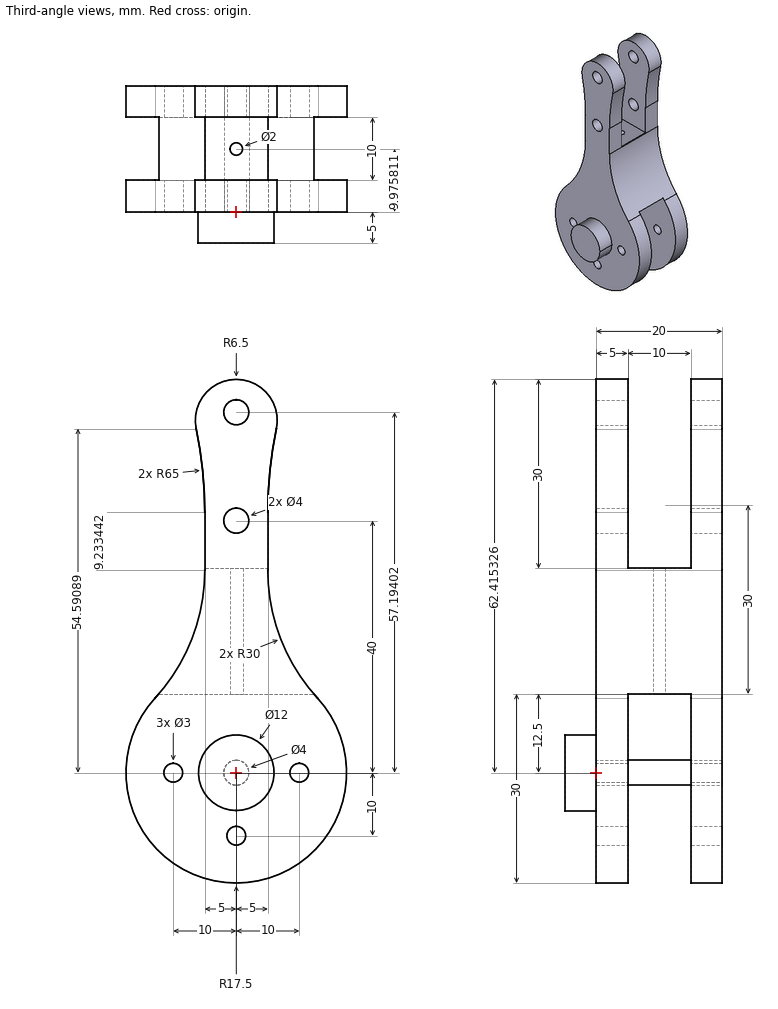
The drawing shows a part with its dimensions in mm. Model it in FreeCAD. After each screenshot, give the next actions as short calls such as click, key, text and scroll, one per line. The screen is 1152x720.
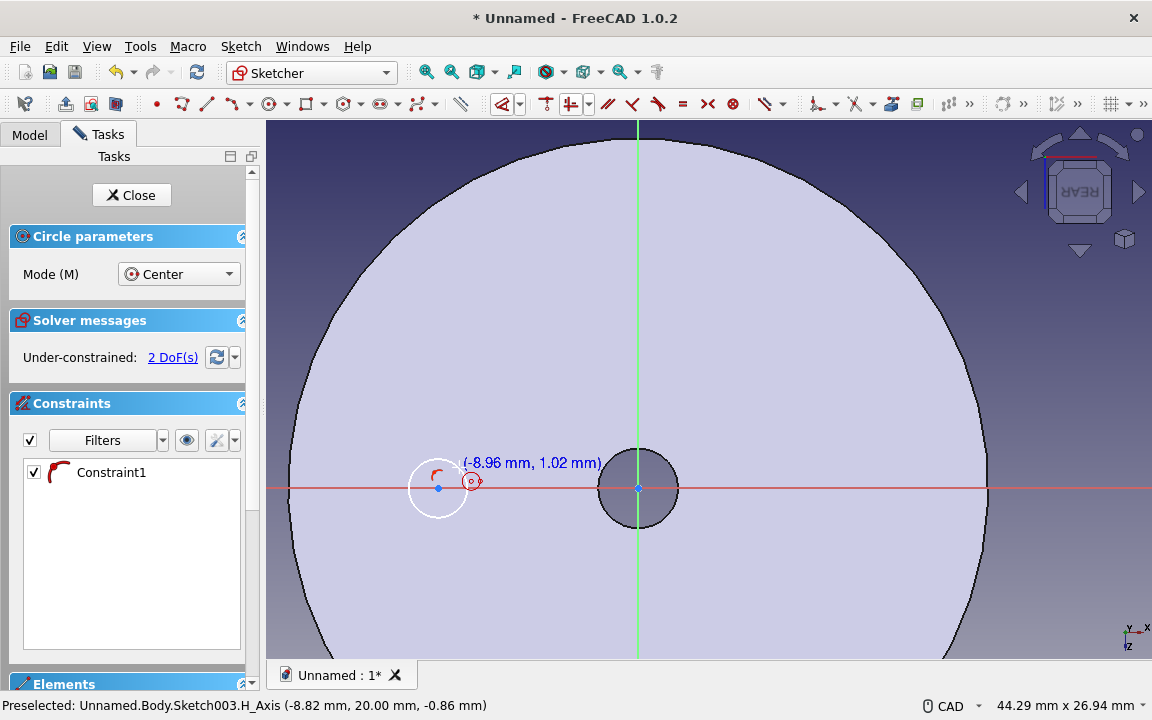
click(838, 488)
click(859, 467)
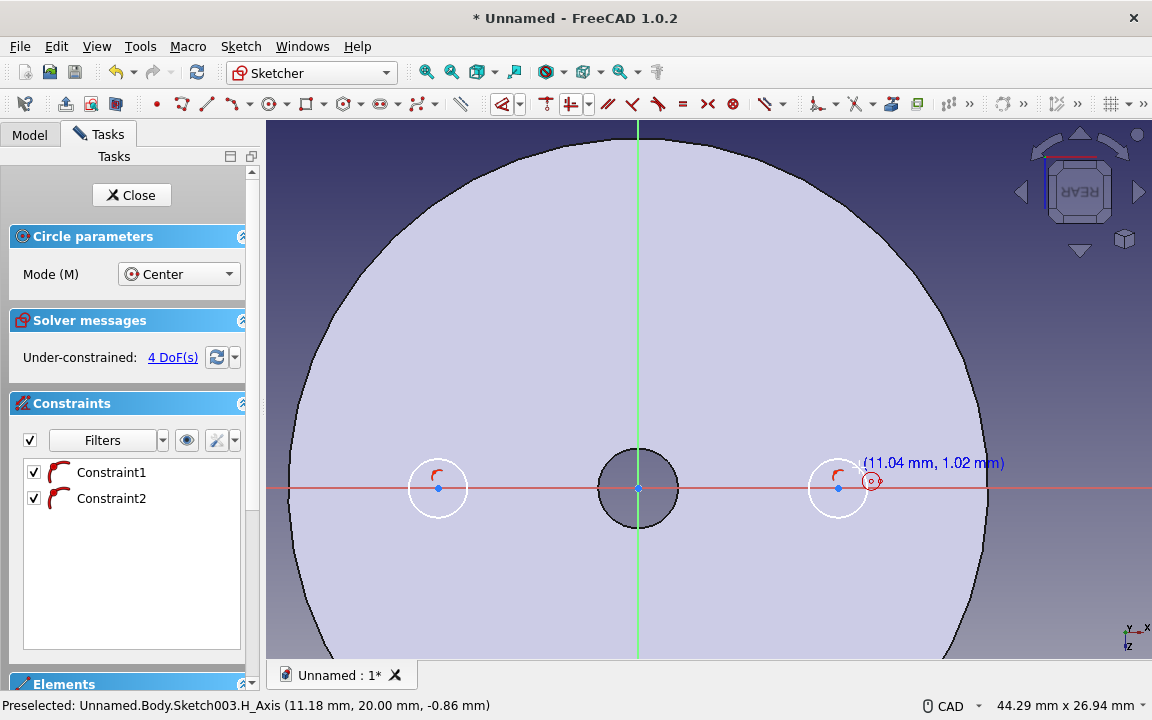
click(638, 288)
click(659, 267)
key(Escape)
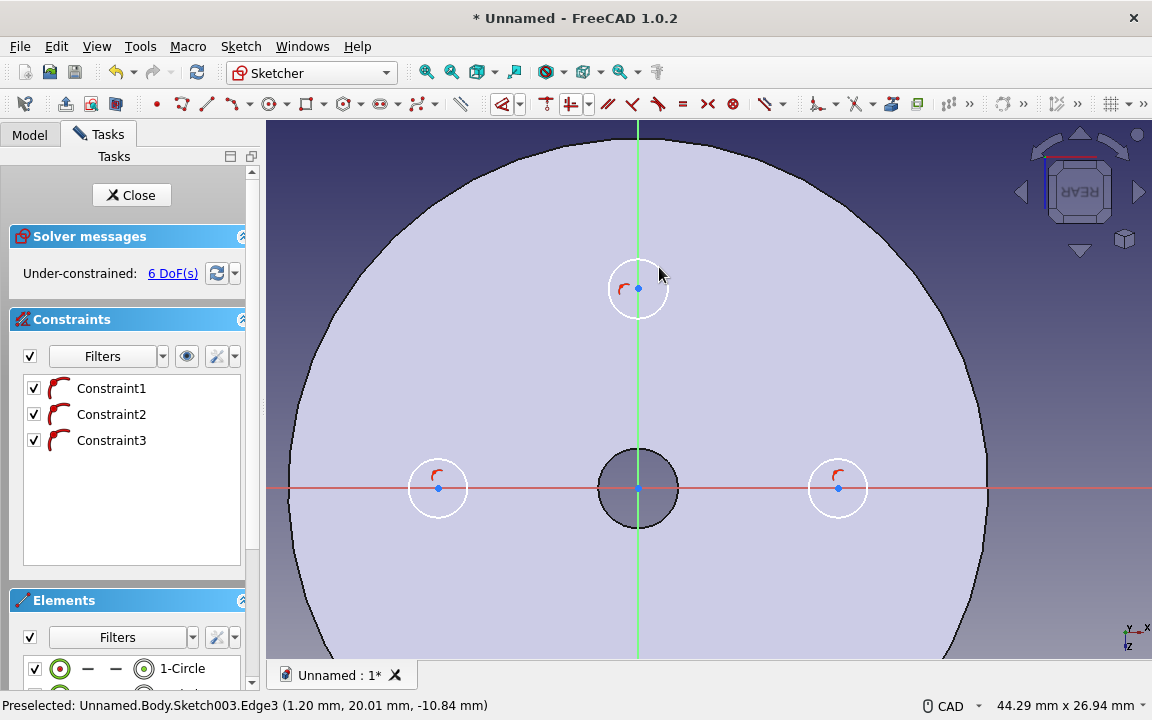
click(459, 468)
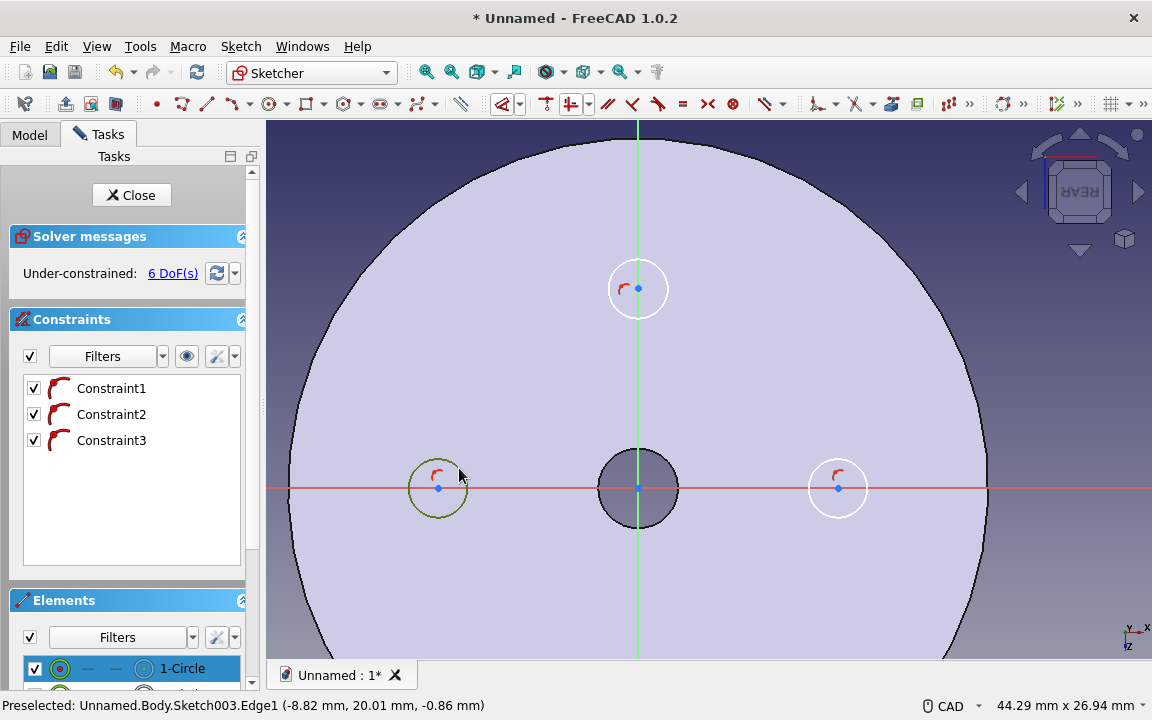
click(859, 468)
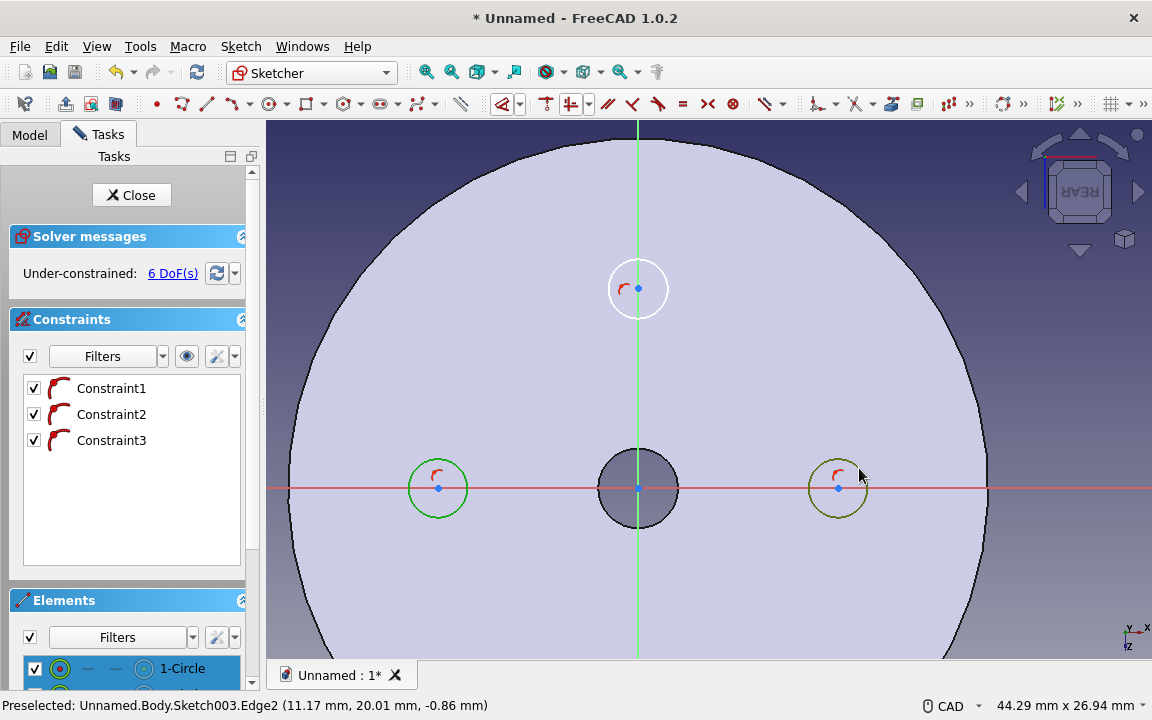
click(659, 268)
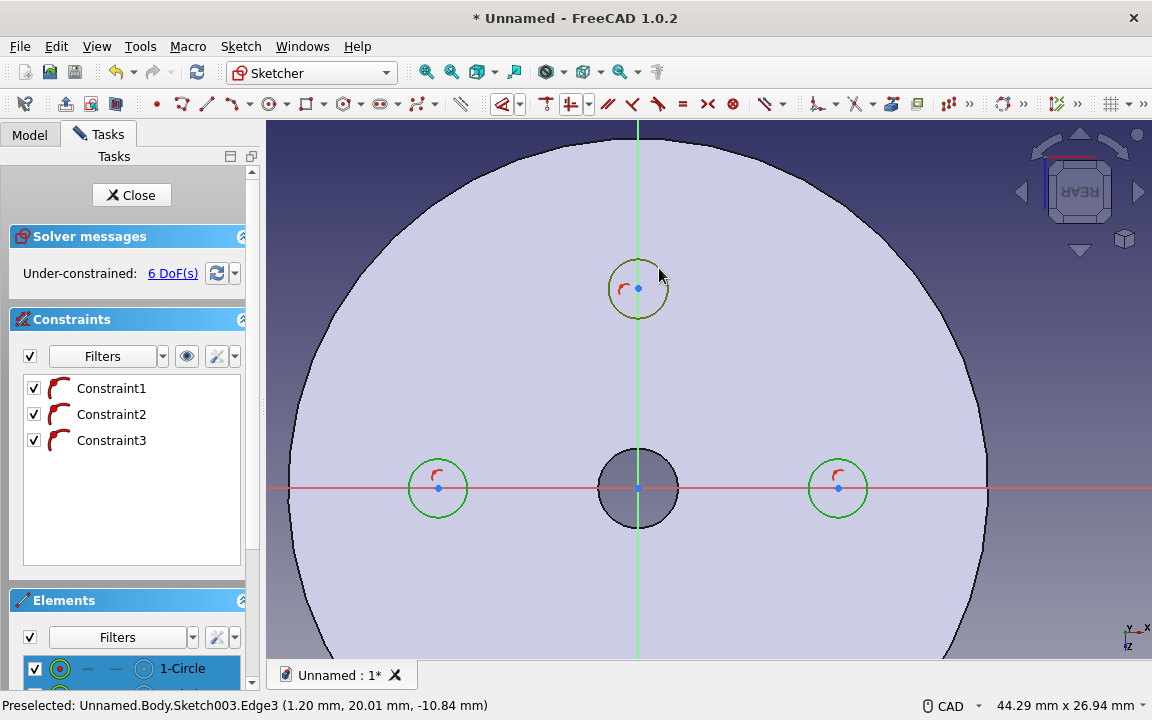
click(683, 104)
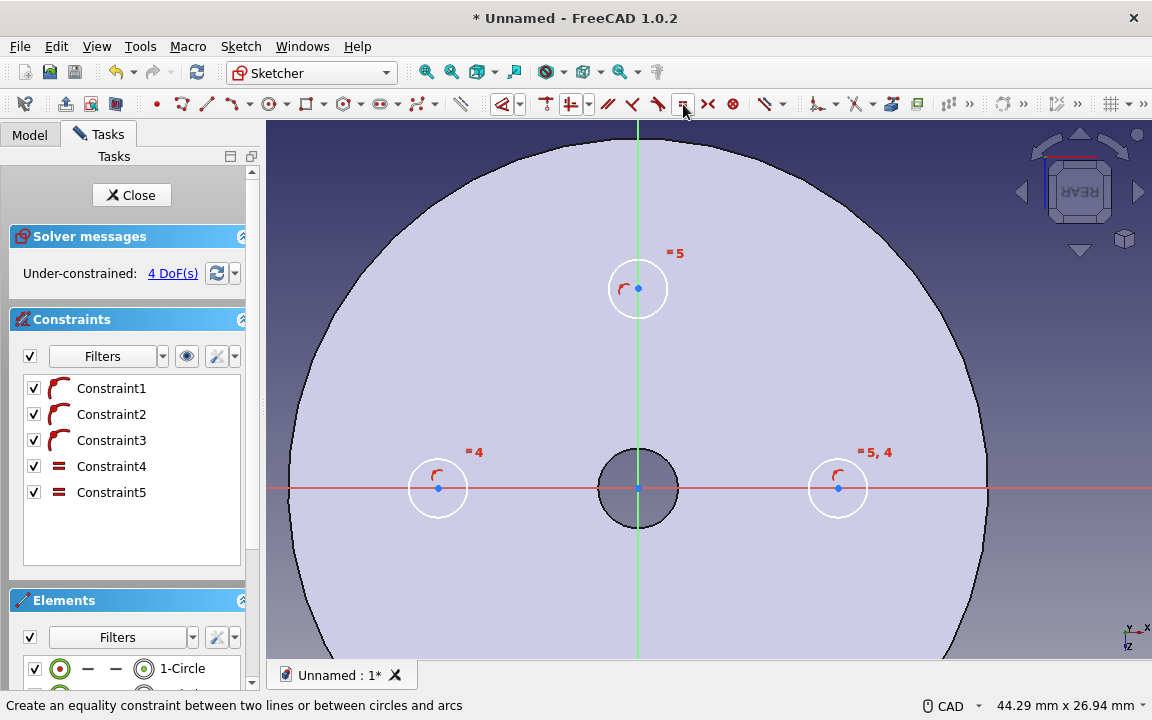
click(459, 468)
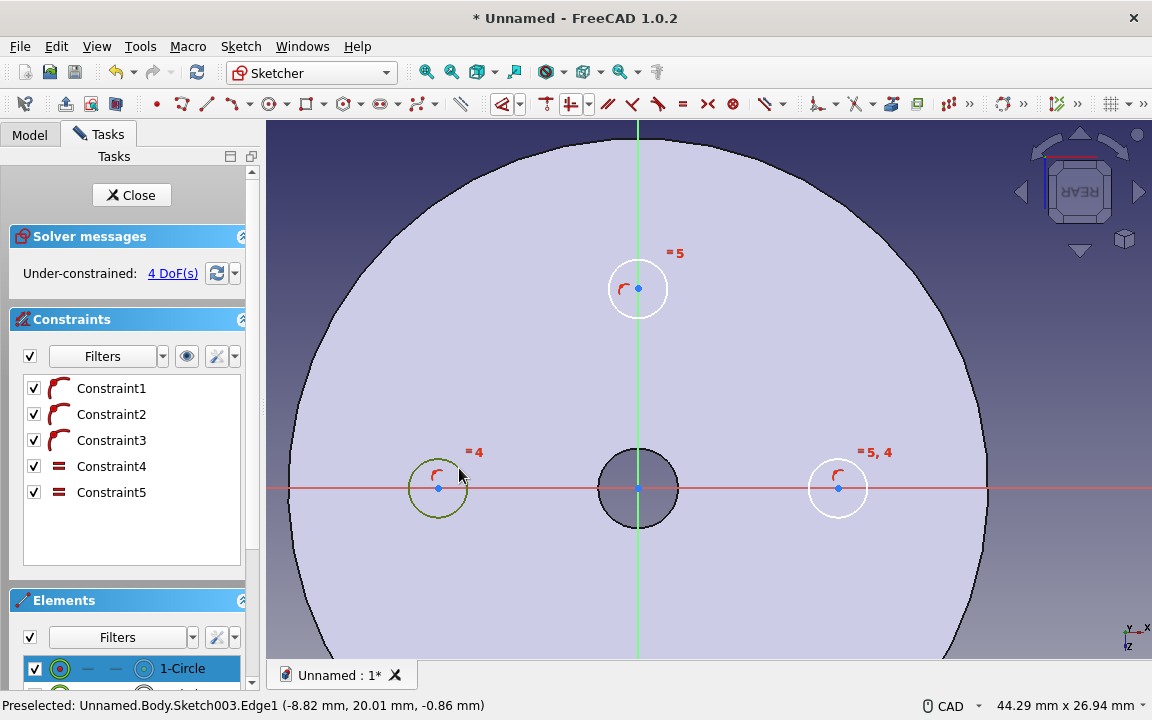
key(k)
key(o)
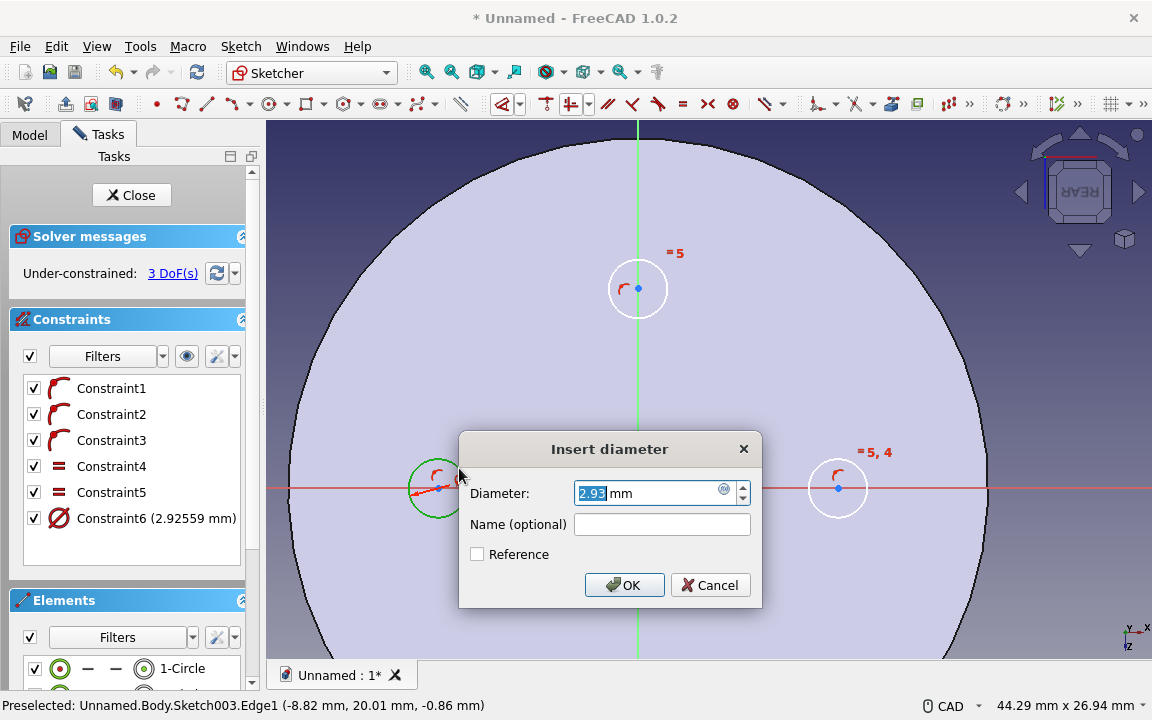
text(3)
key(Return)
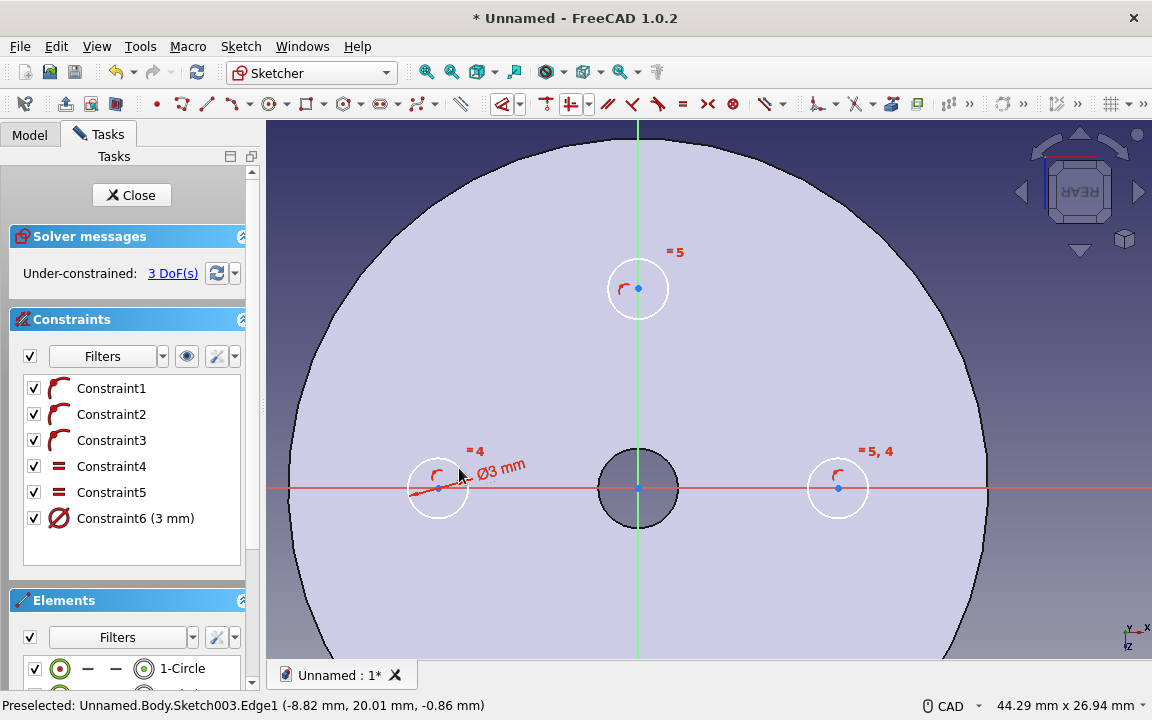
click(438, 488)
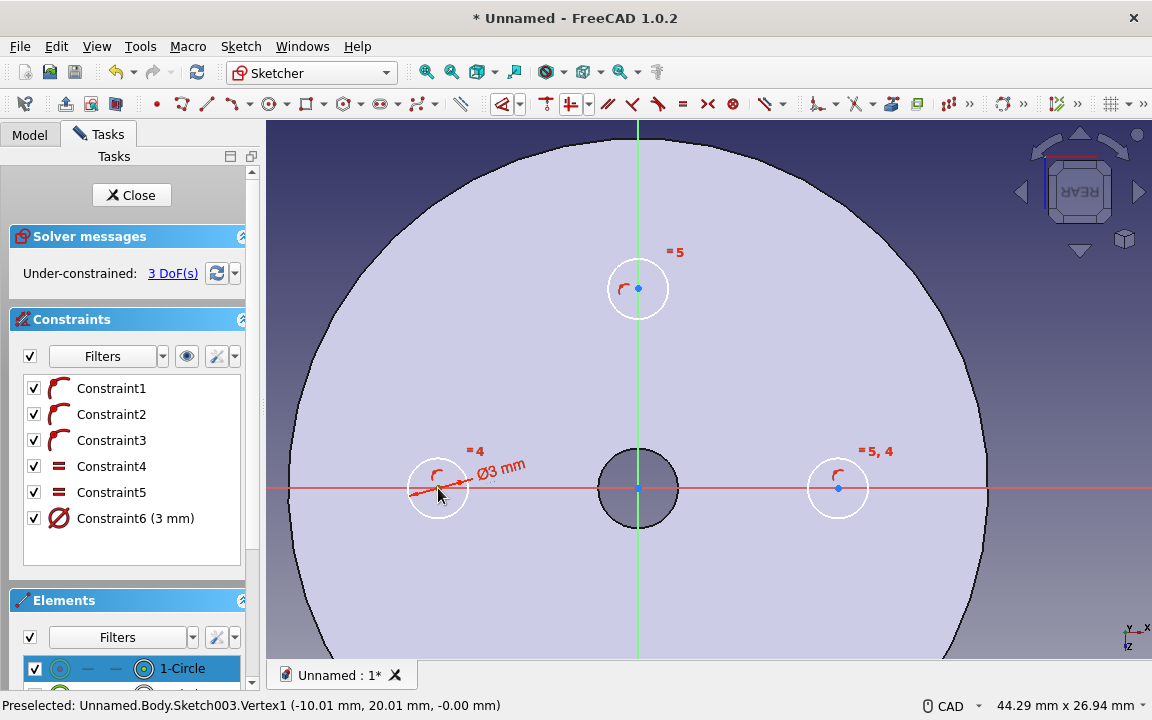
click(520, 104)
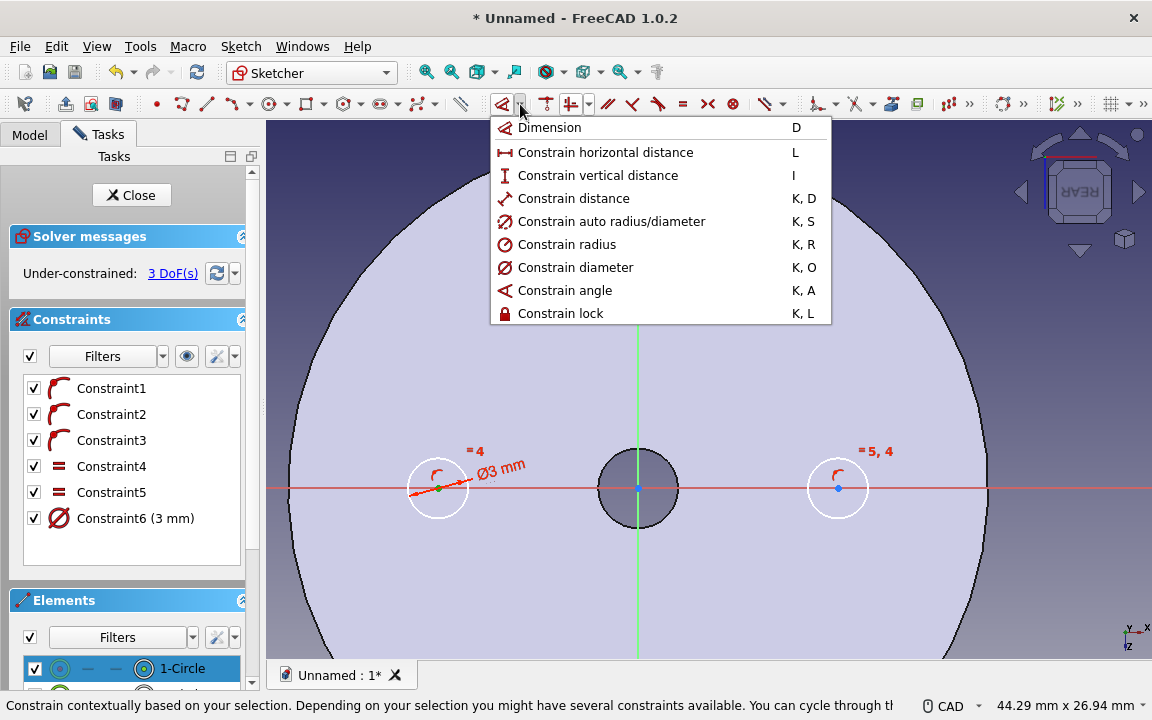
click(661, 152)